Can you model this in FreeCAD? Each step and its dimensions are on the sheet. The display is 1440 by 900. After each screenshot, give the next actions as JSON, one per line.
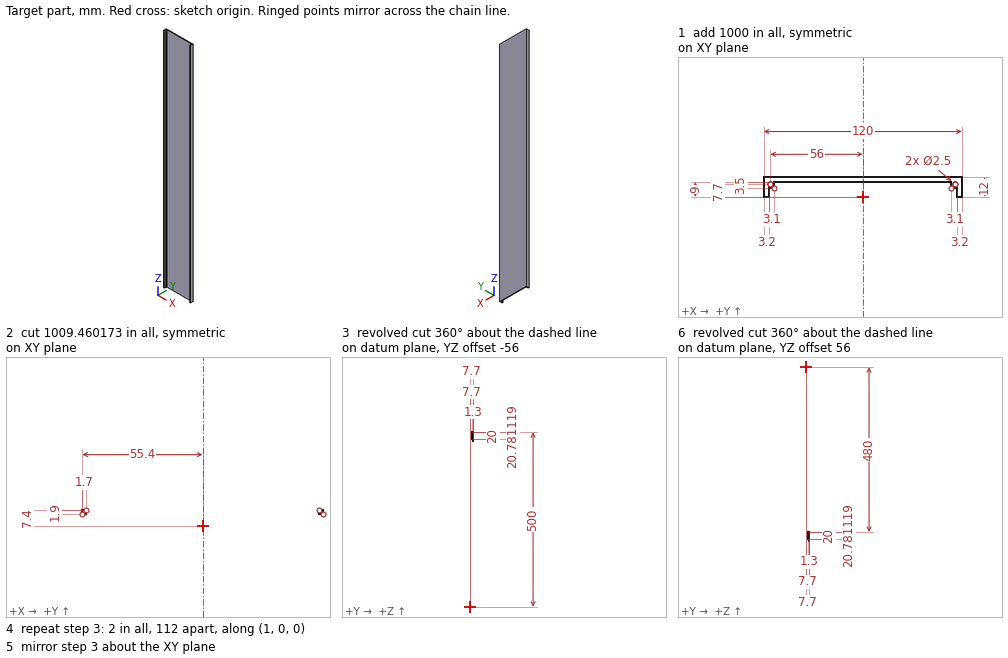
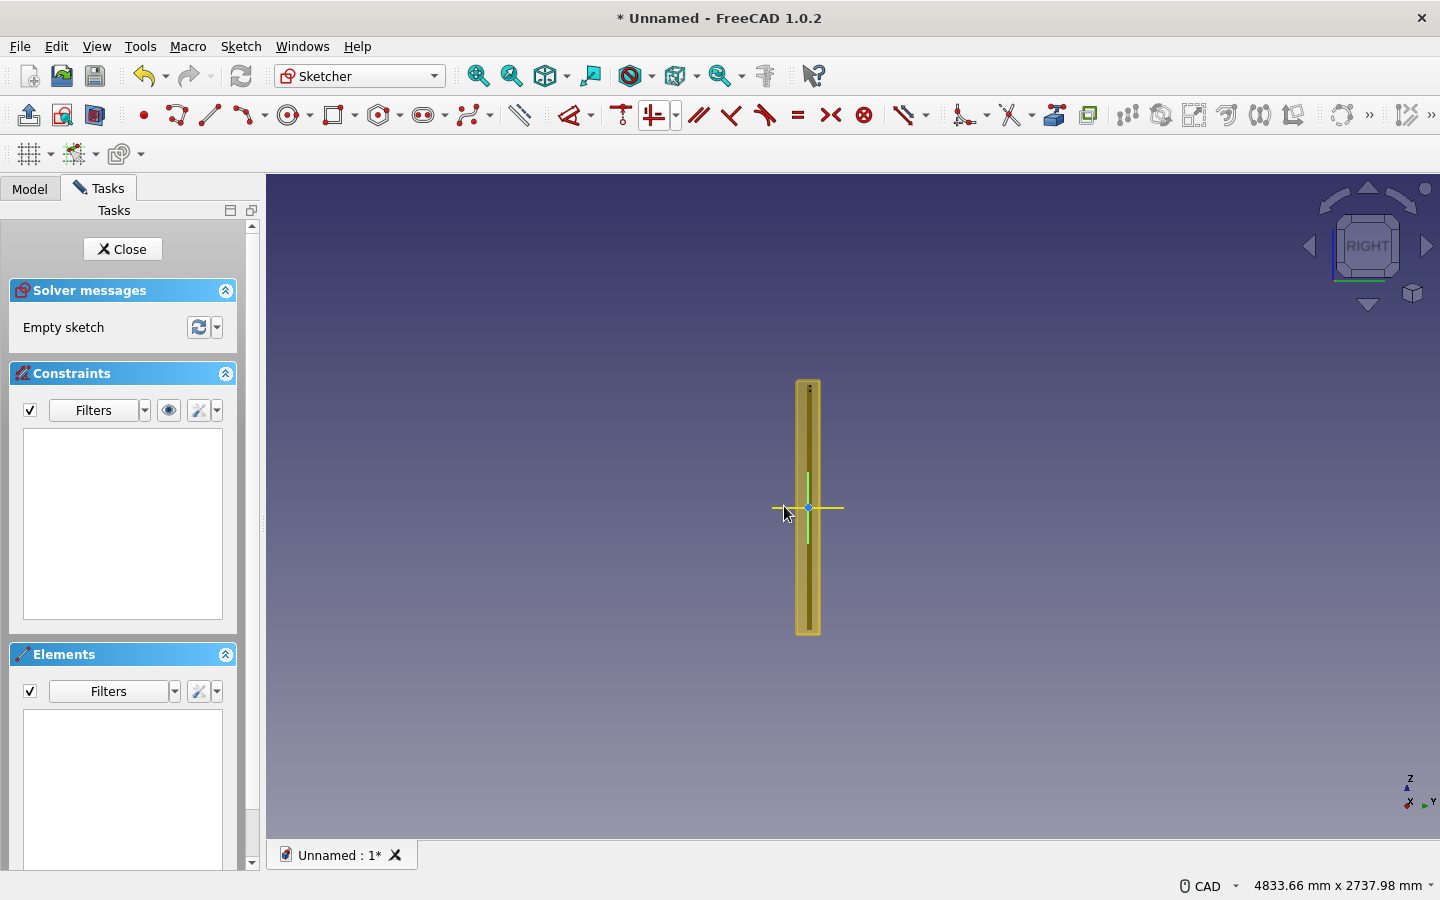
{"action": "scroll", "coordinate": [811, 634], "scroll_direction": "up", "scroll_amount": 15}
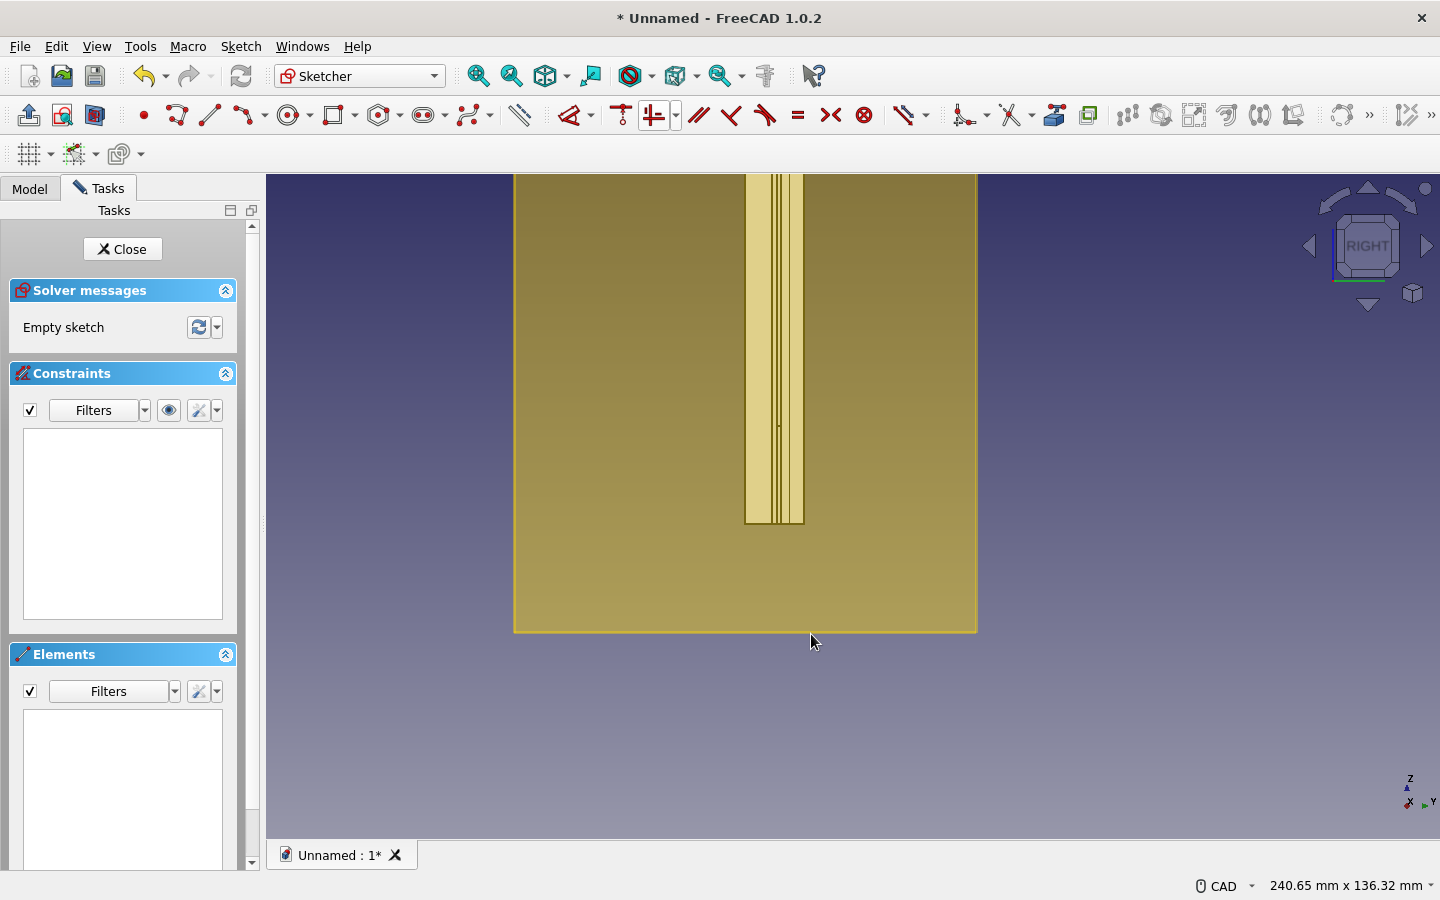
{"action": "scroll", "coordinate": [777, 487], "scroll_direction": "up", "scroll_amount": 6}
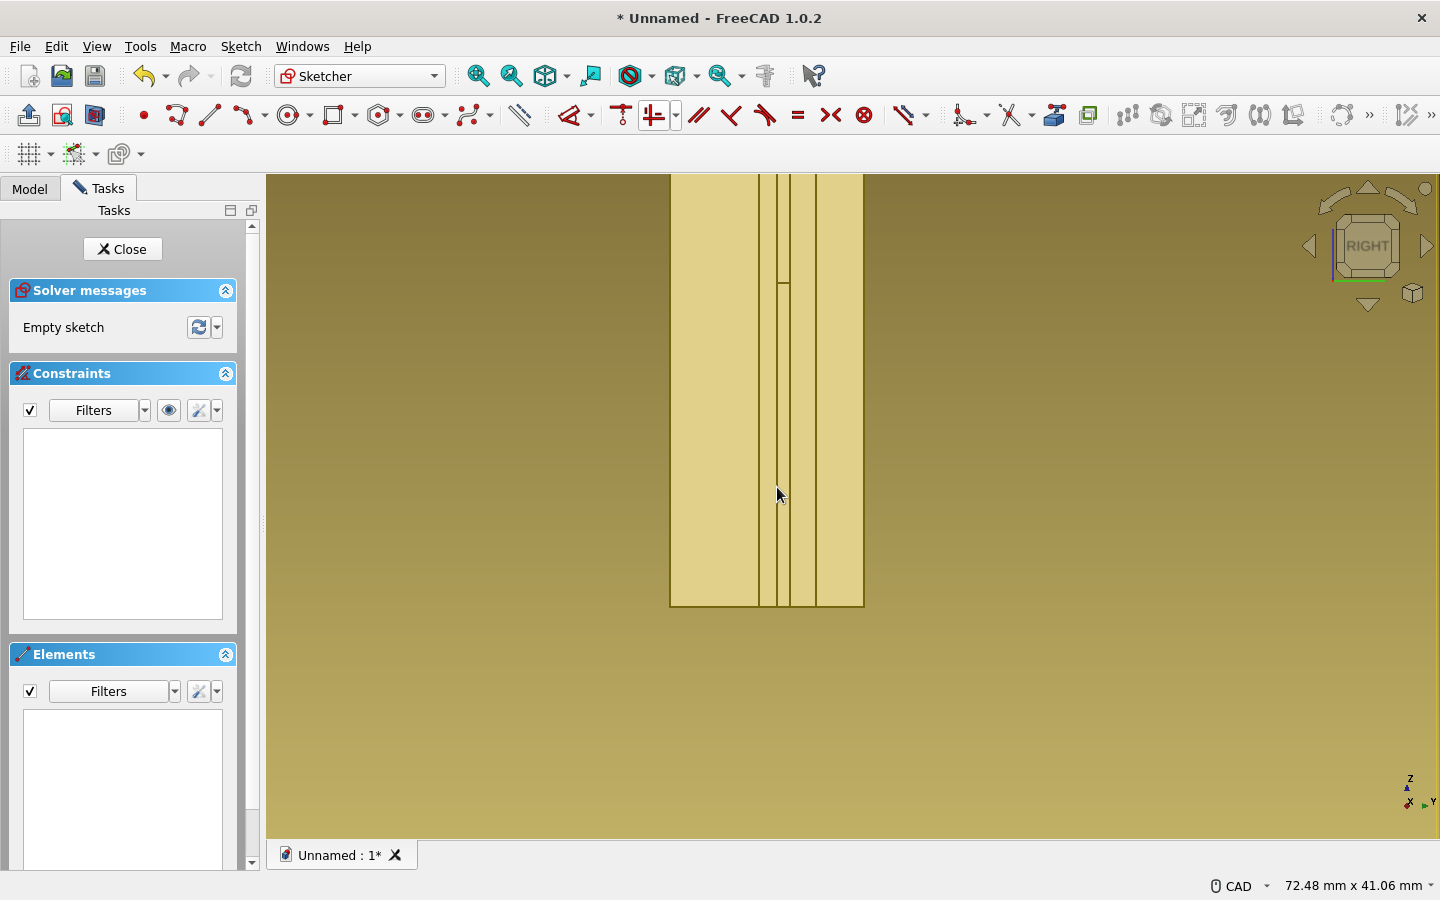
{"action": "key", "text": "g m"}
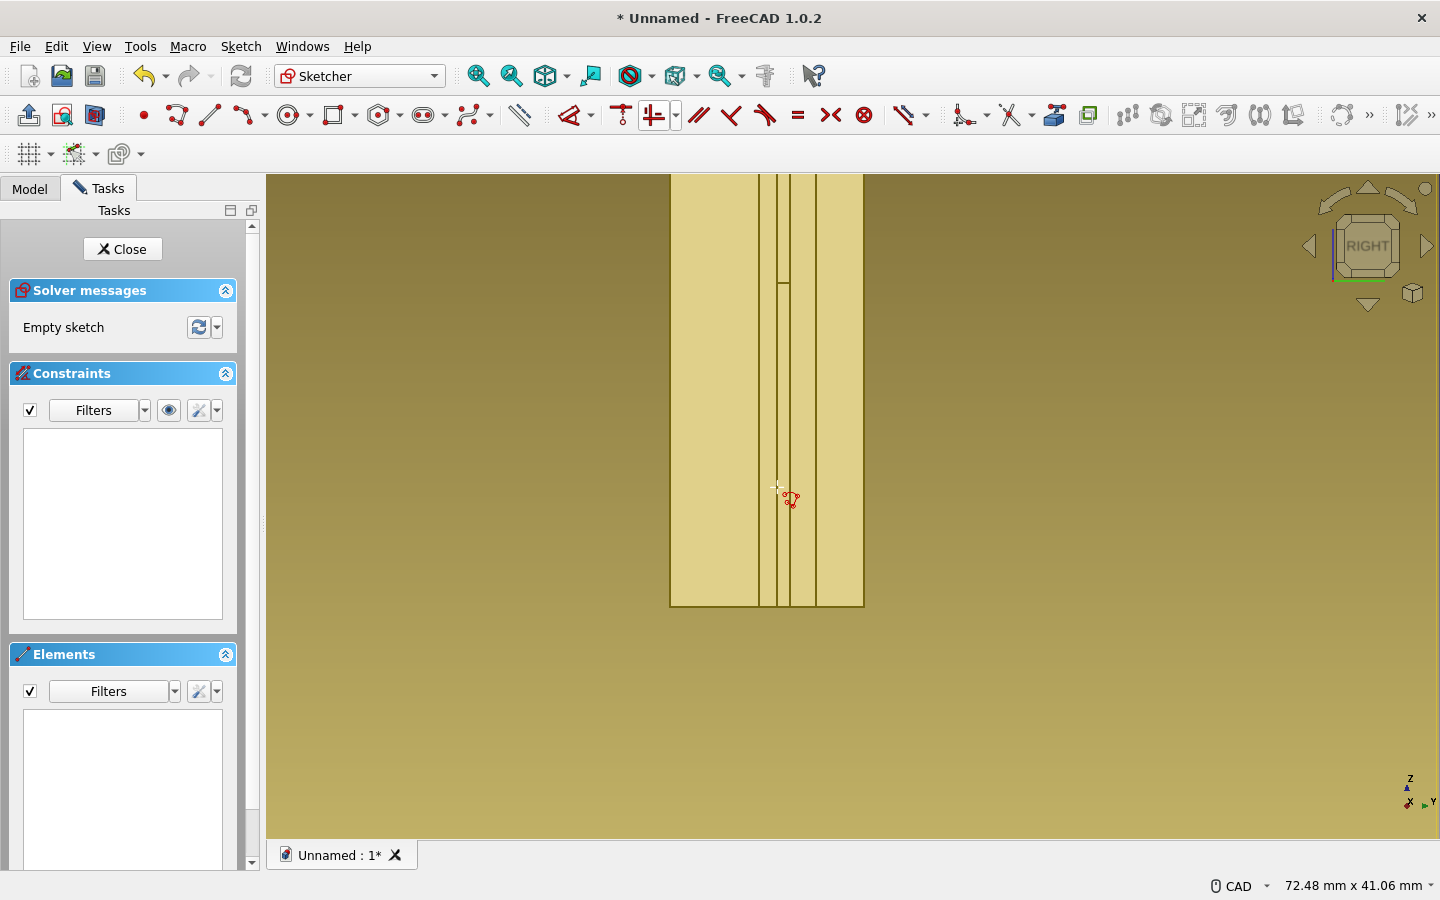
{"action": "left_click", "coordinate": [795, 271]}
{"action": "left_click", "coordinate": [774, 283]}
{"action": "left_click", "coordinate": [774, 607]}
{"action": "left_click", "coordinate": [795, 607]}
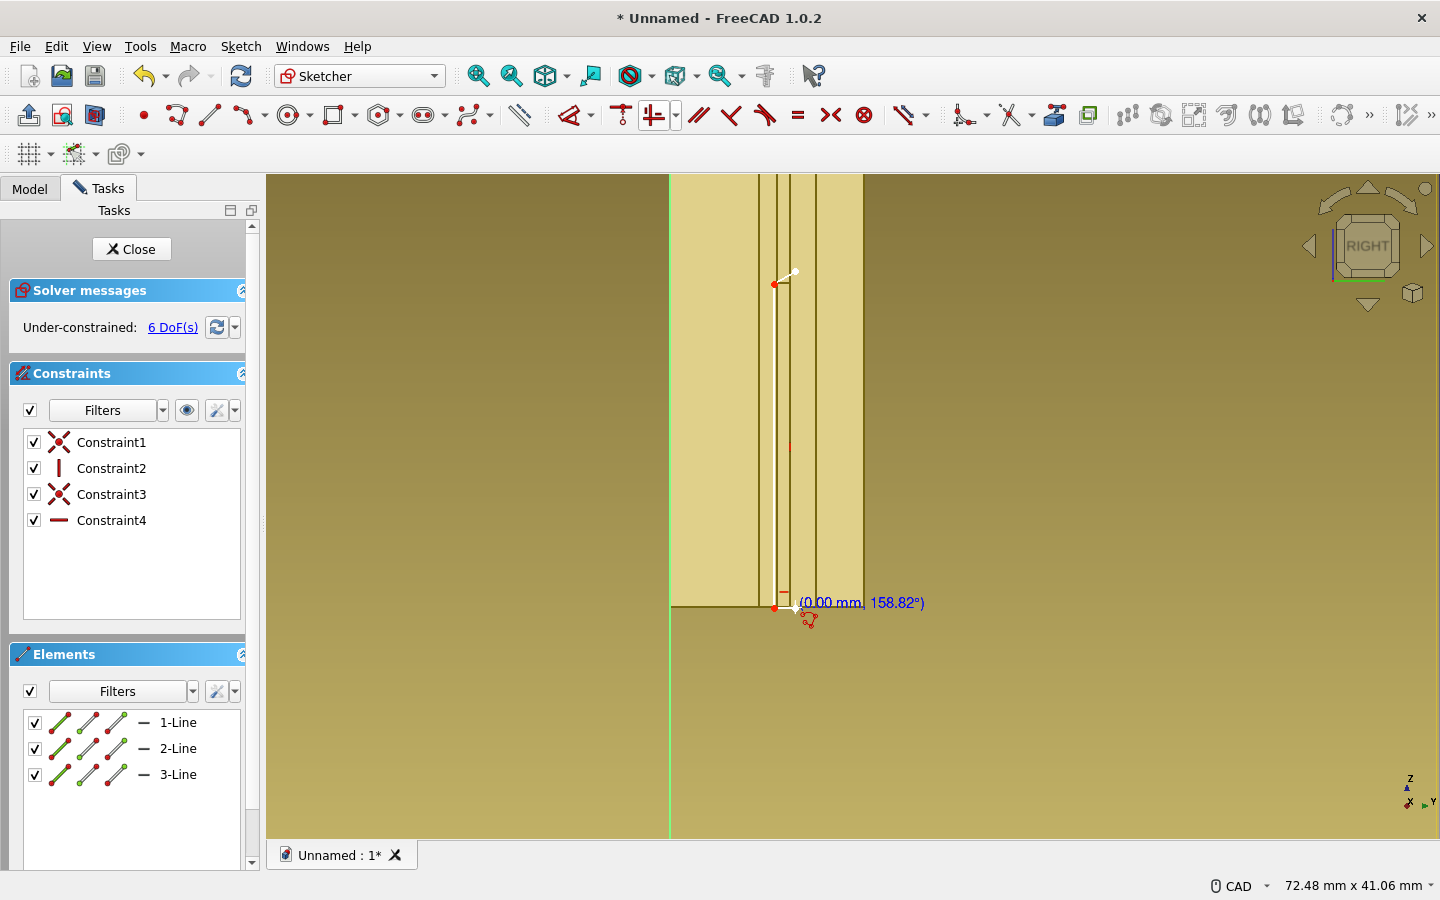
{"action": "scroll", "coordinate": [795, 271], "scroll_direction": "up", "scroll_amount": 2}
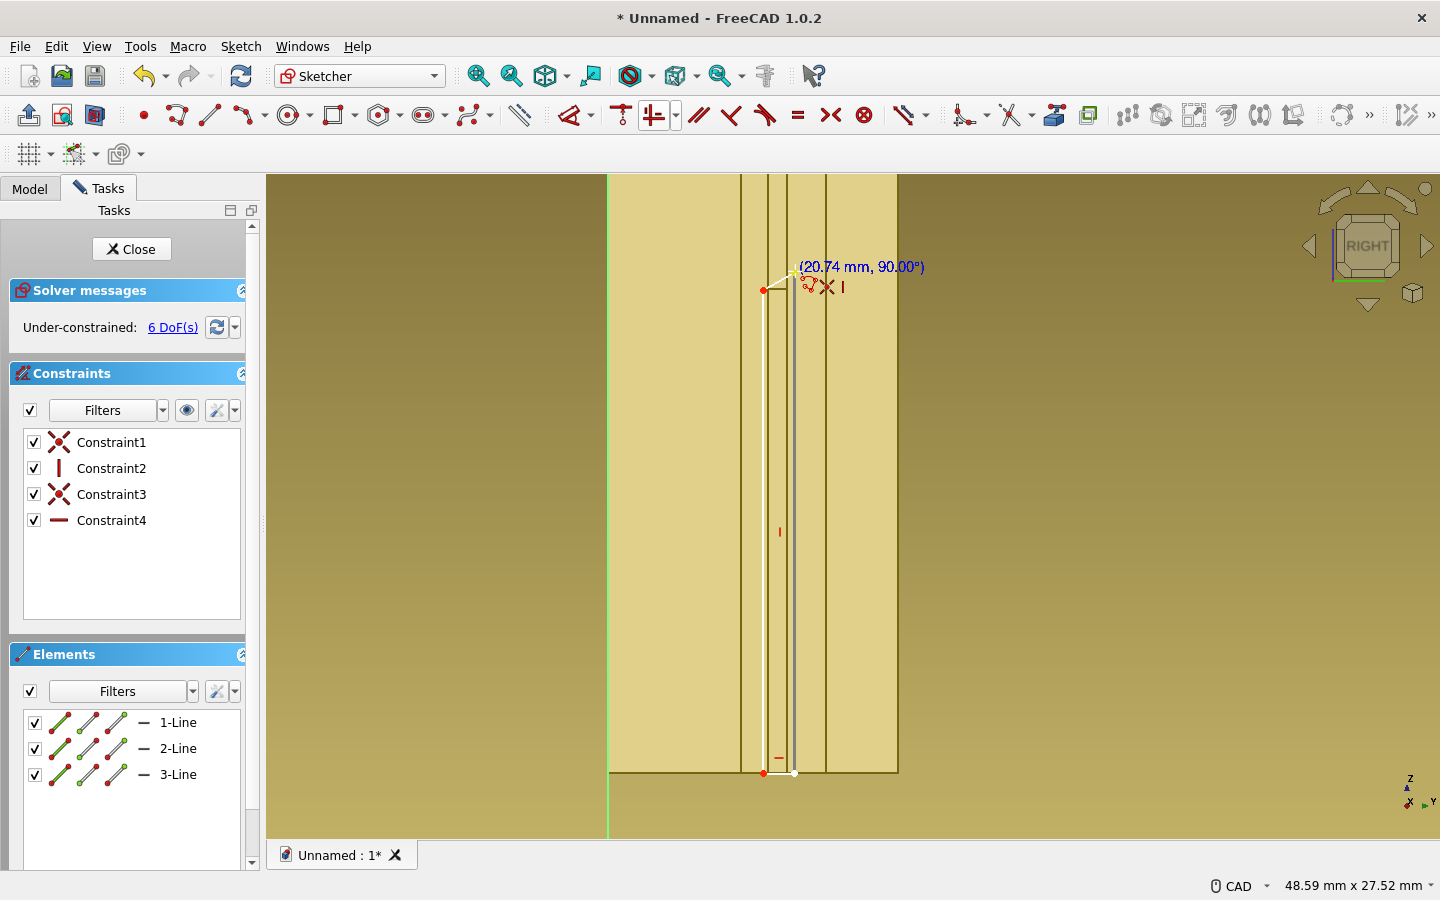
{"action": "left_click", "coordinate": [795, 272]}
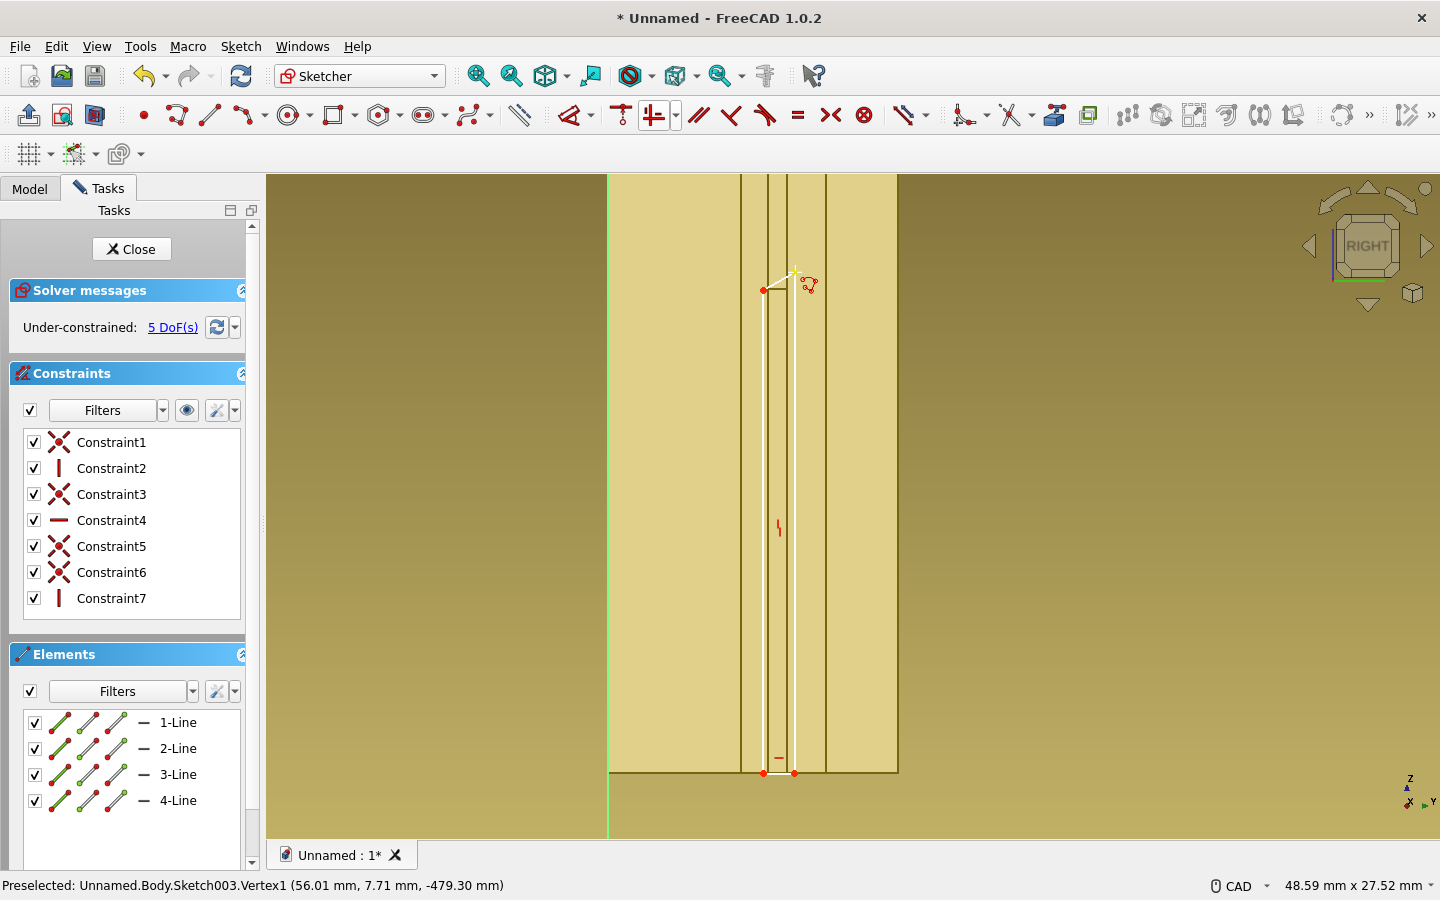
{"action": "key", "text": "g l"}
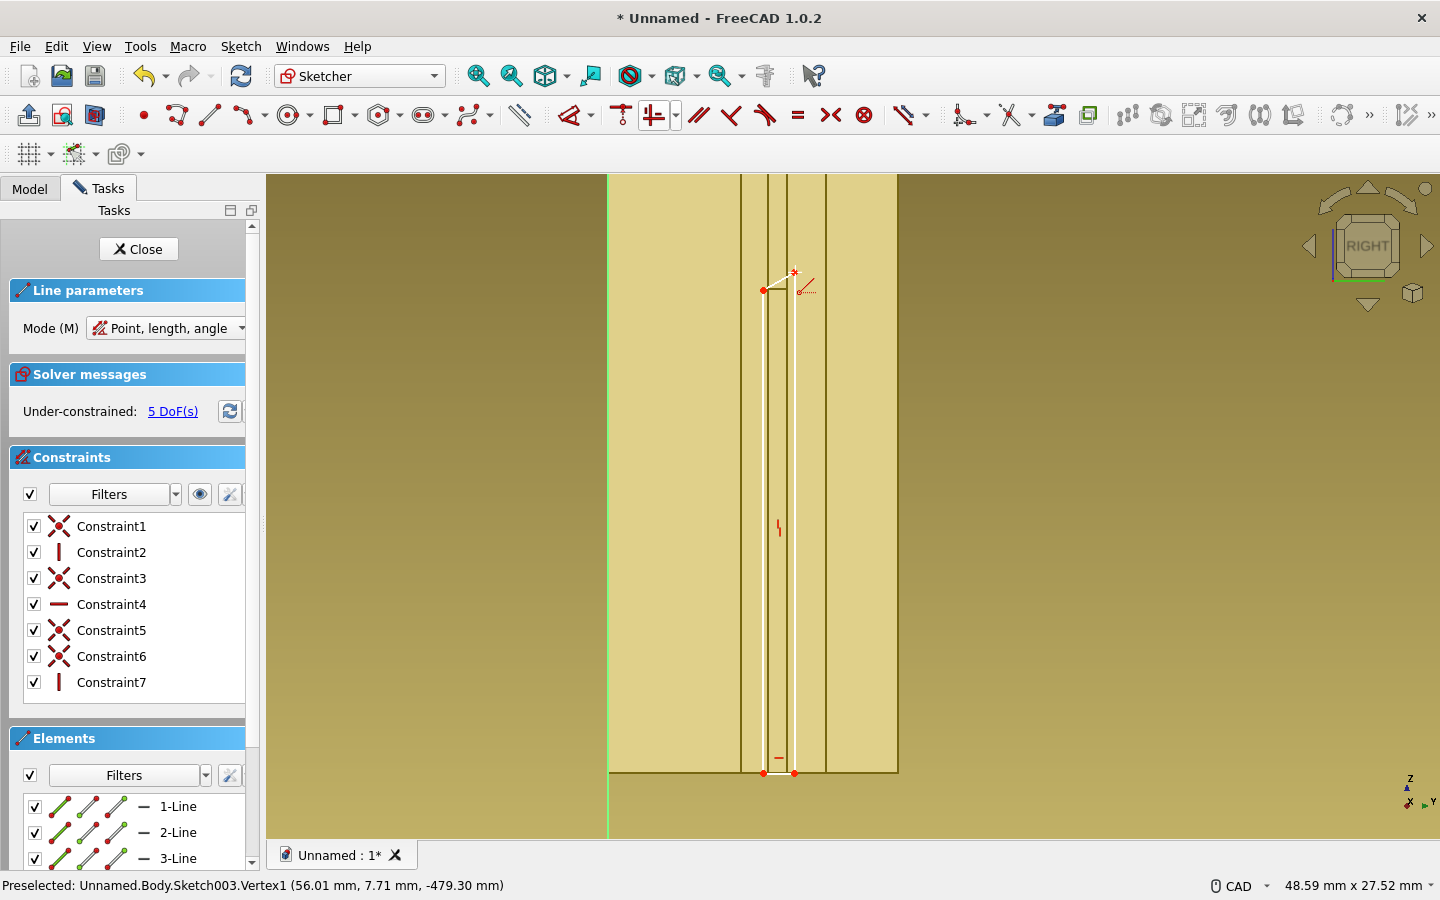
{"action": "scroll", "coordinate": [796, 272], "scroll_direction": "down", "scroll_amount": 2}